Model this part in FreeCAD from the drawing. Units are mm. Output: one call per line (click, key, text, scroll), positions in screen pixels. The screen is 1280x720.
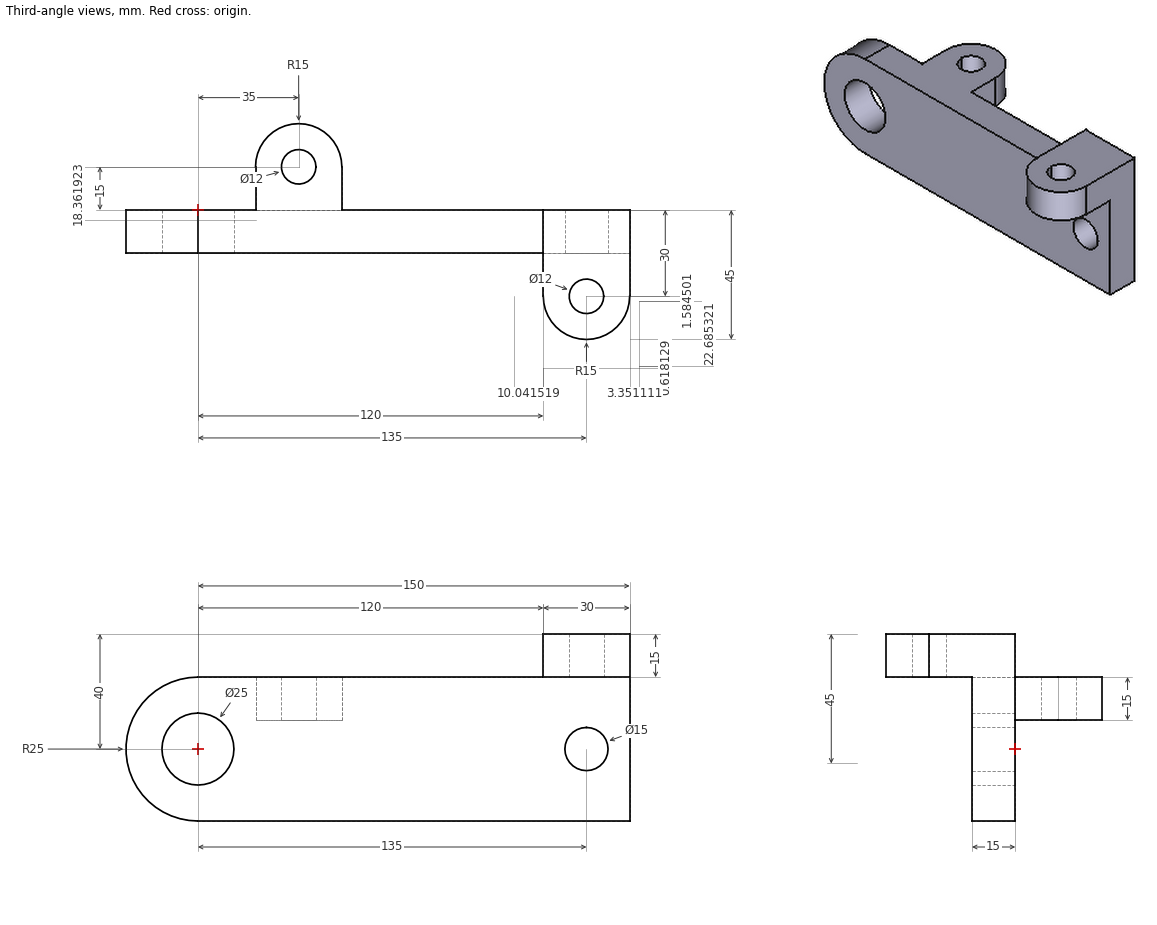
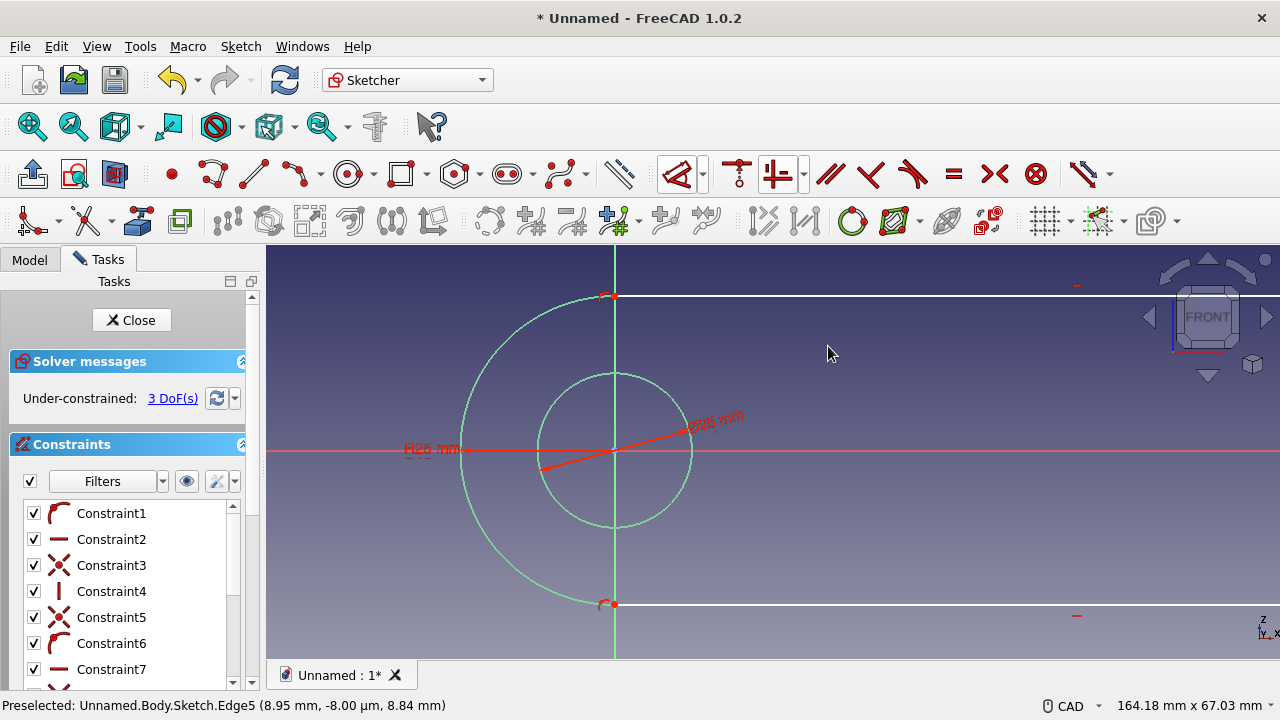
scroll(344, 454, down, 3)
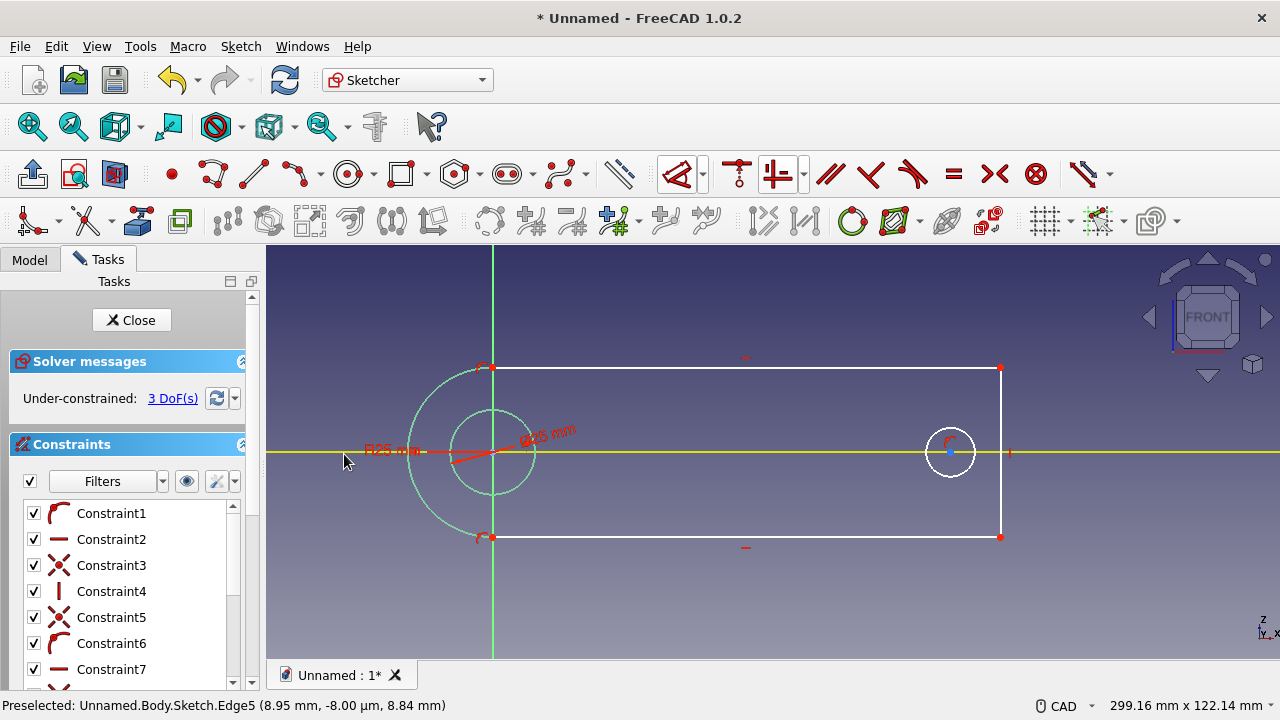
click(968, 435)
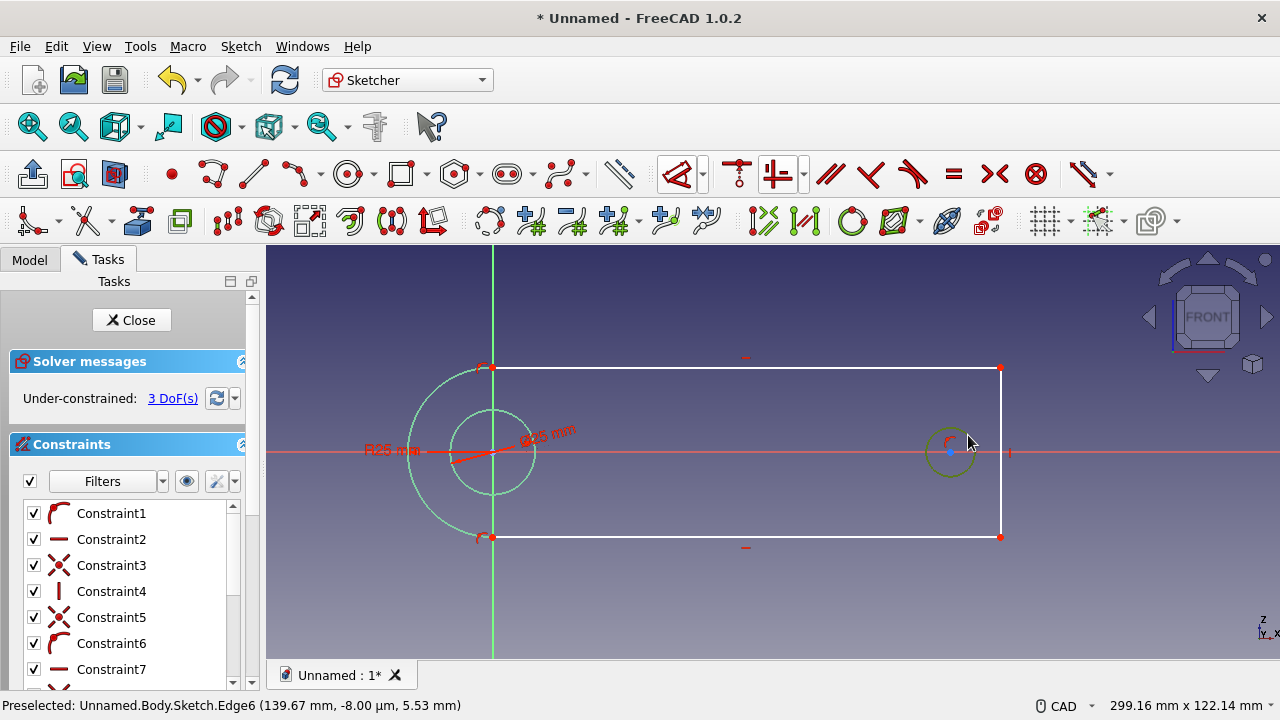
click(702, 174)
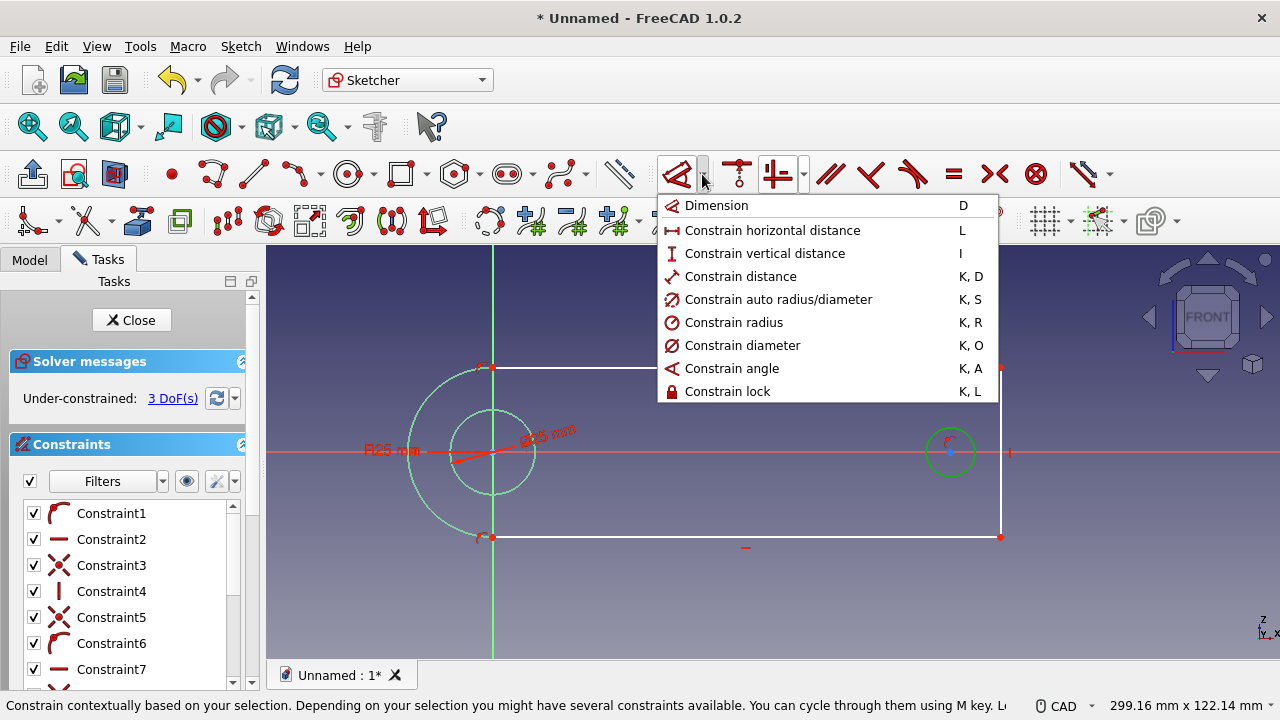
click(828, 346)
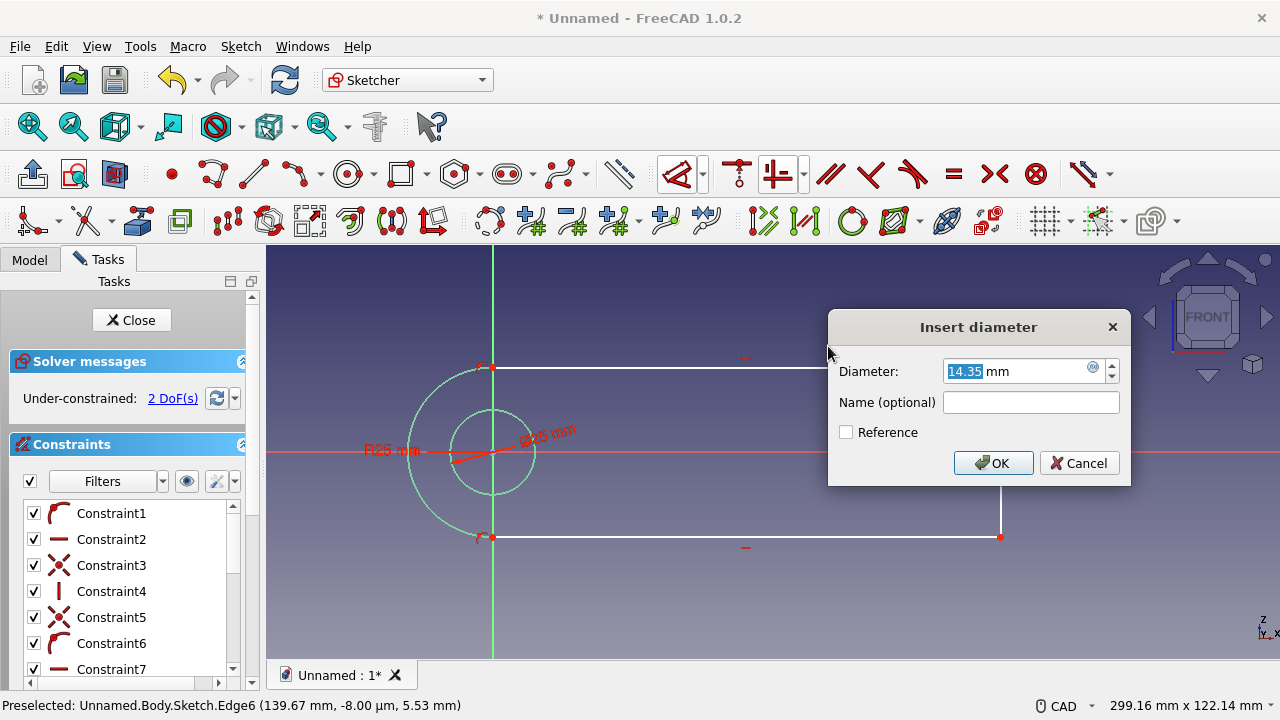
text(15)
key(Return)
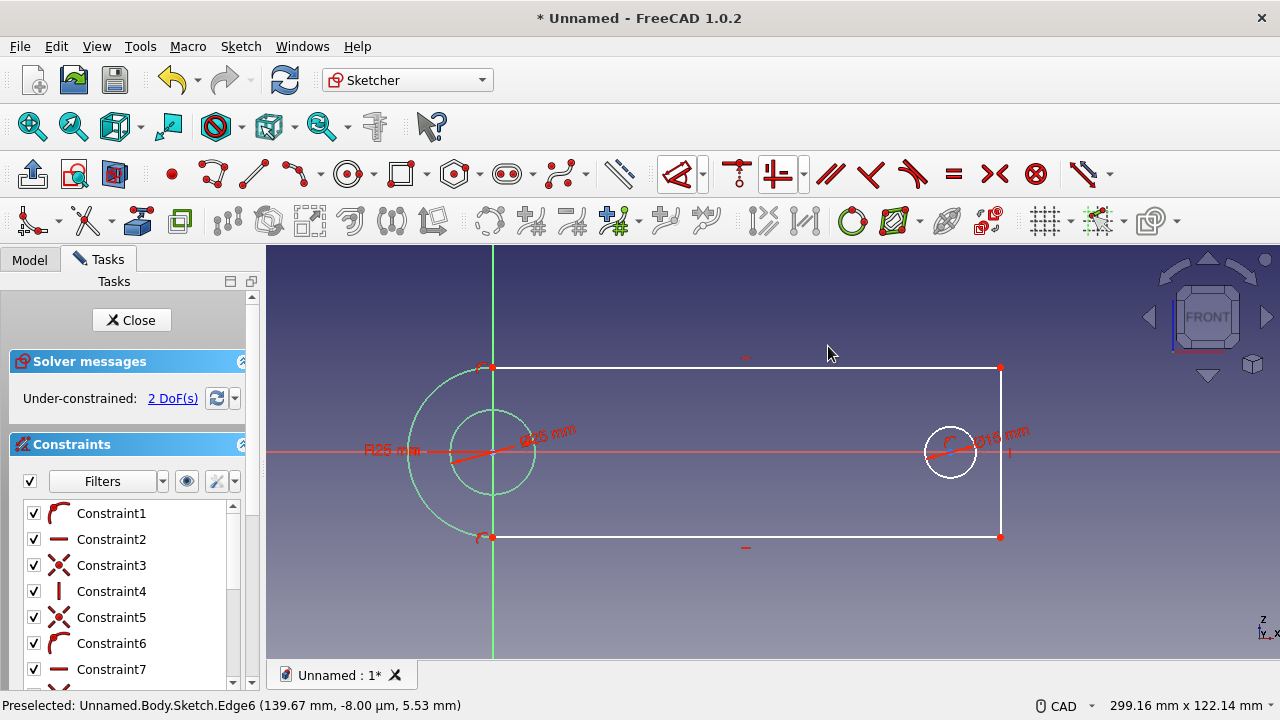
click(645, 368)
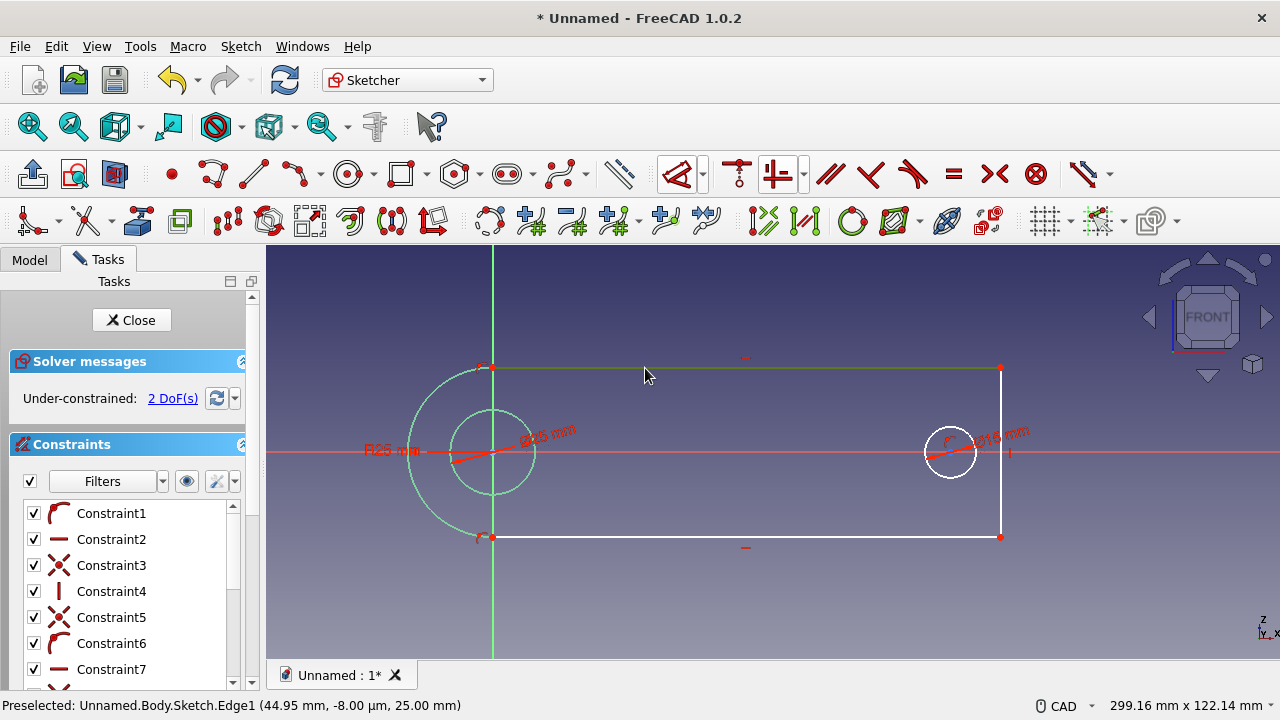
click(702, 174)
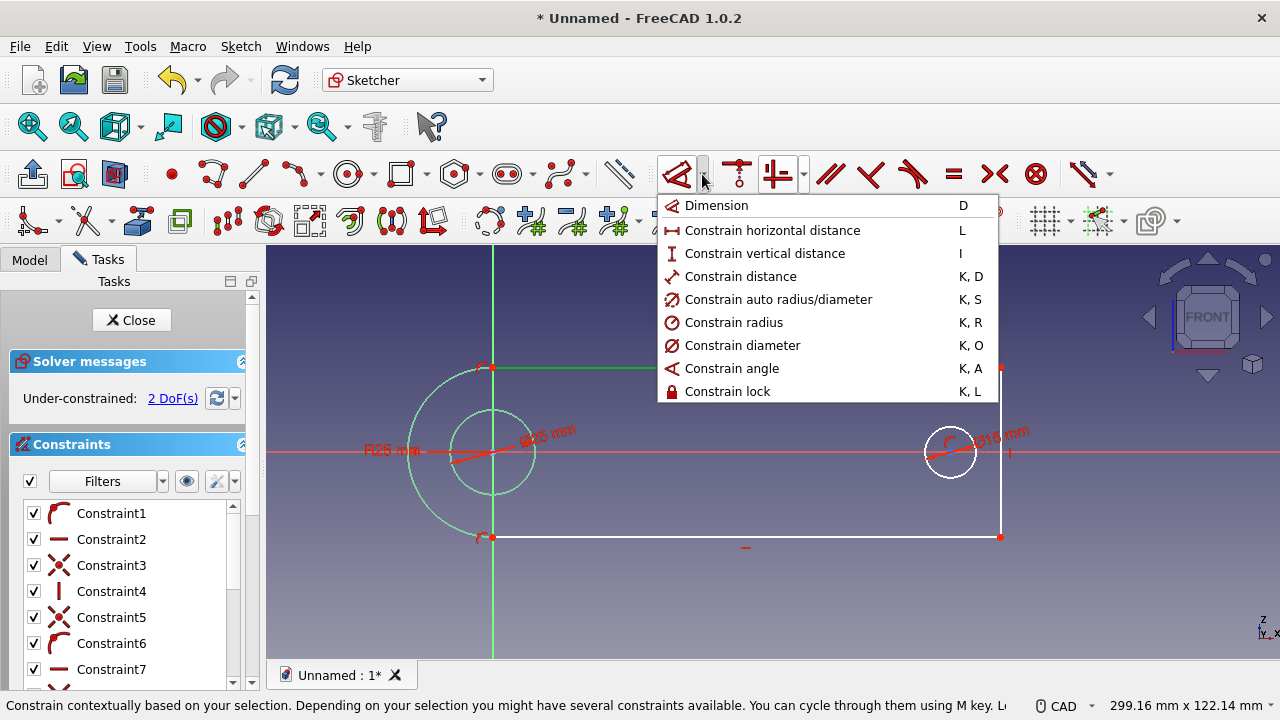
click(828, 230)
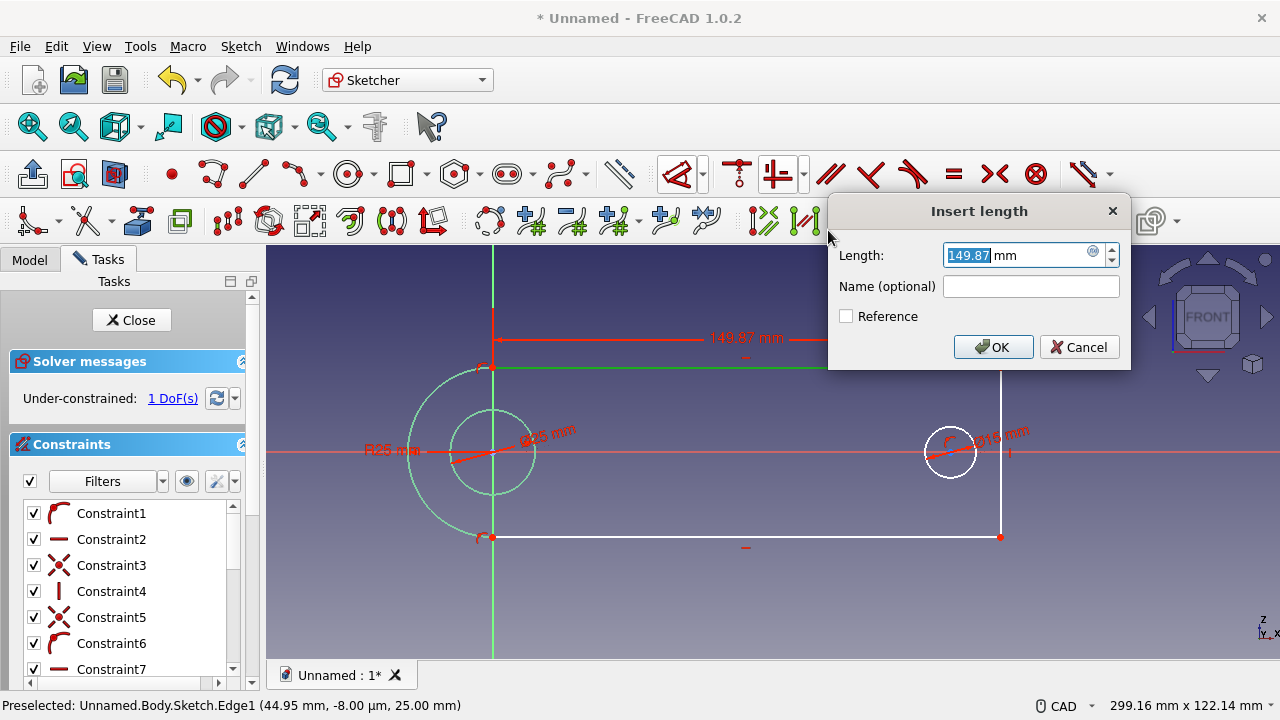
text(150)
key(Return)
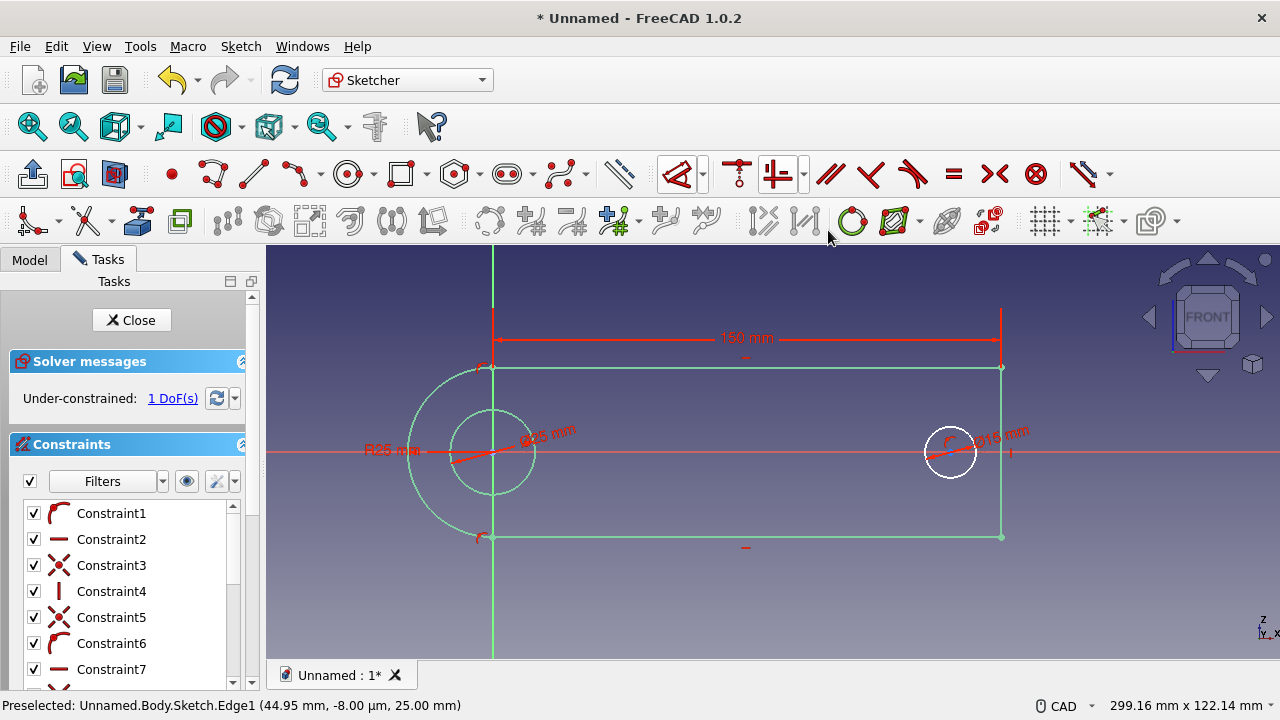
click(951, 452)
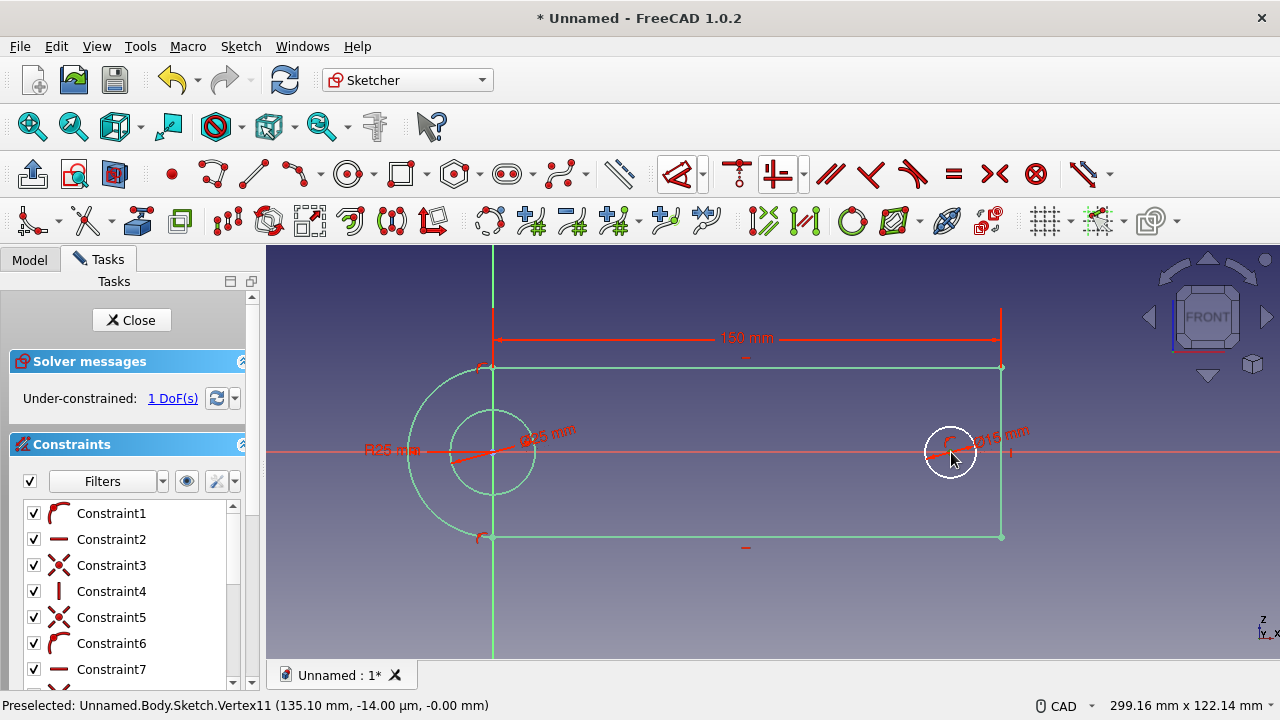
click(702, 174)